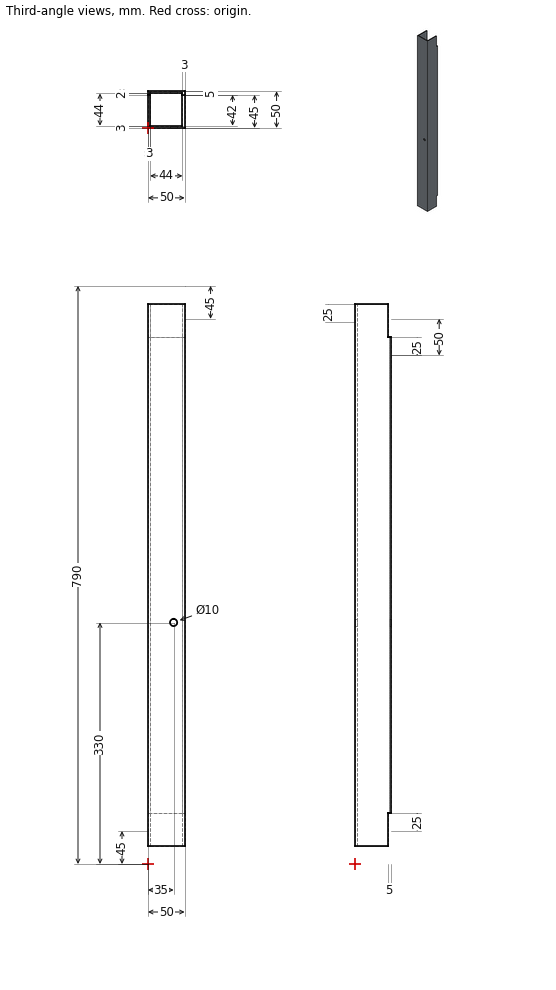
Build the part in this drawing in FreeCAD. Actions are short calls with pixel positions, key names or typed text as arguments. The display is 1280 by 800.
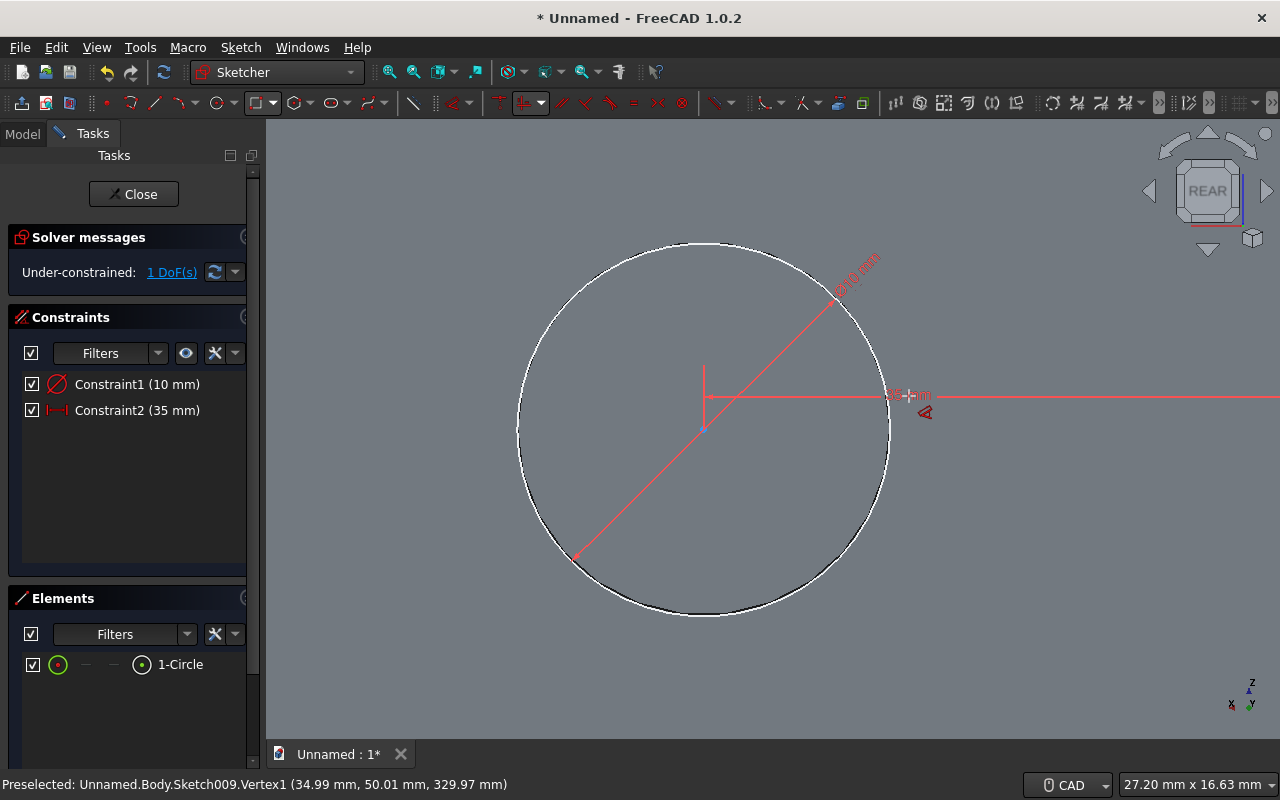
click(704, 430)
click(670, 571)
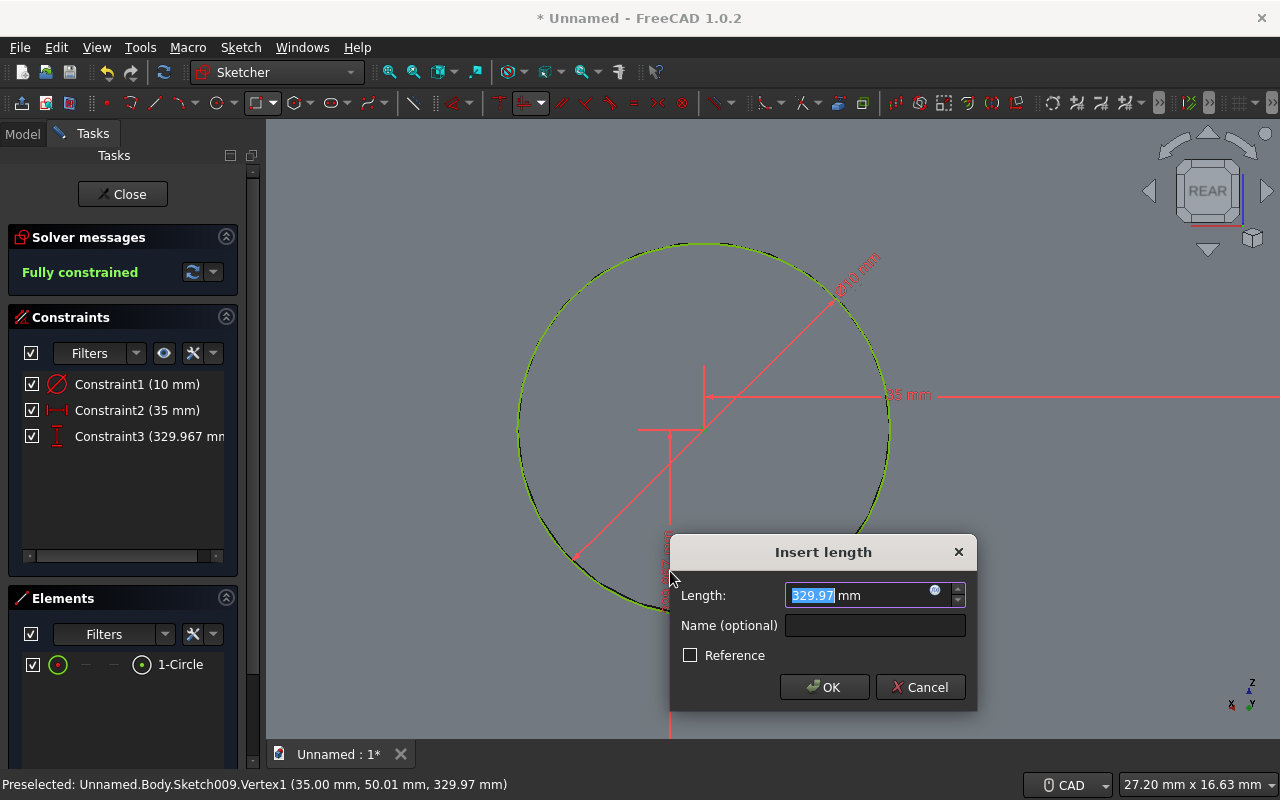
text(330)
key(Return)
key(Escape)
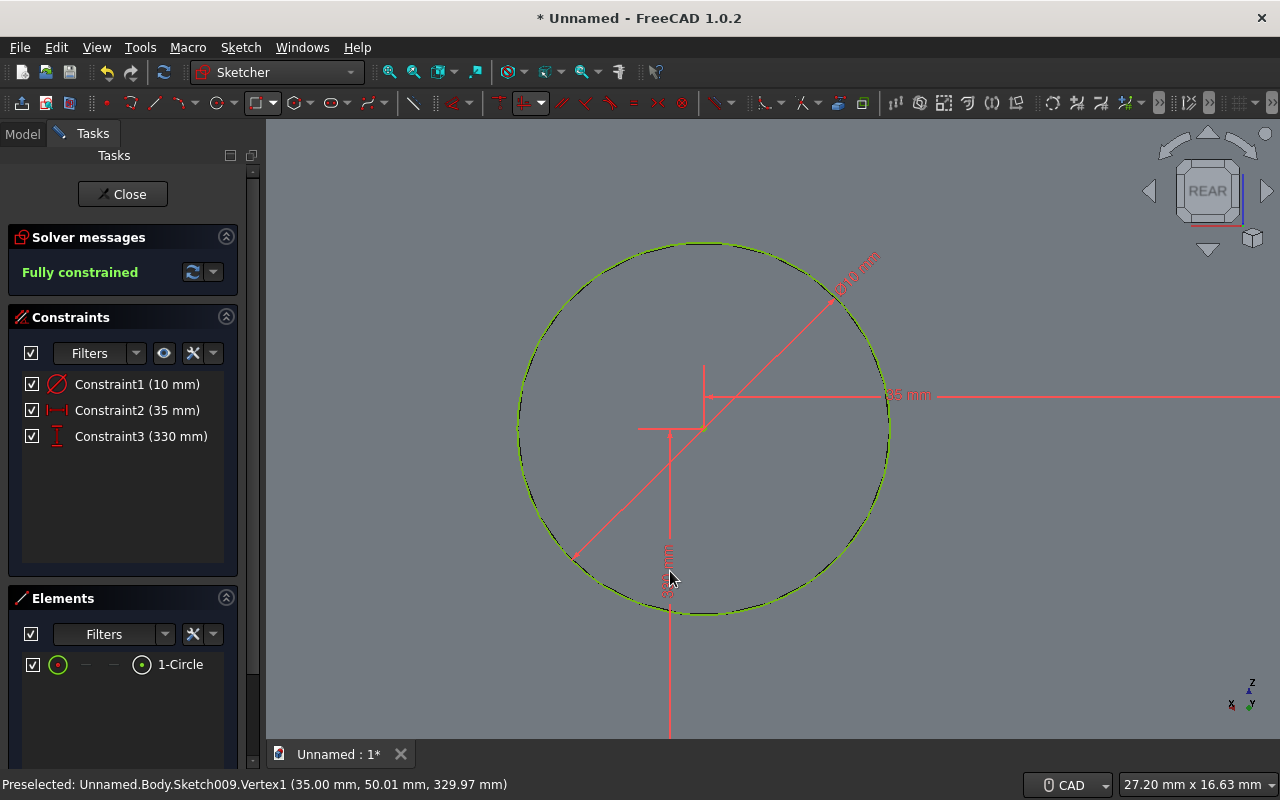
click(123, 194)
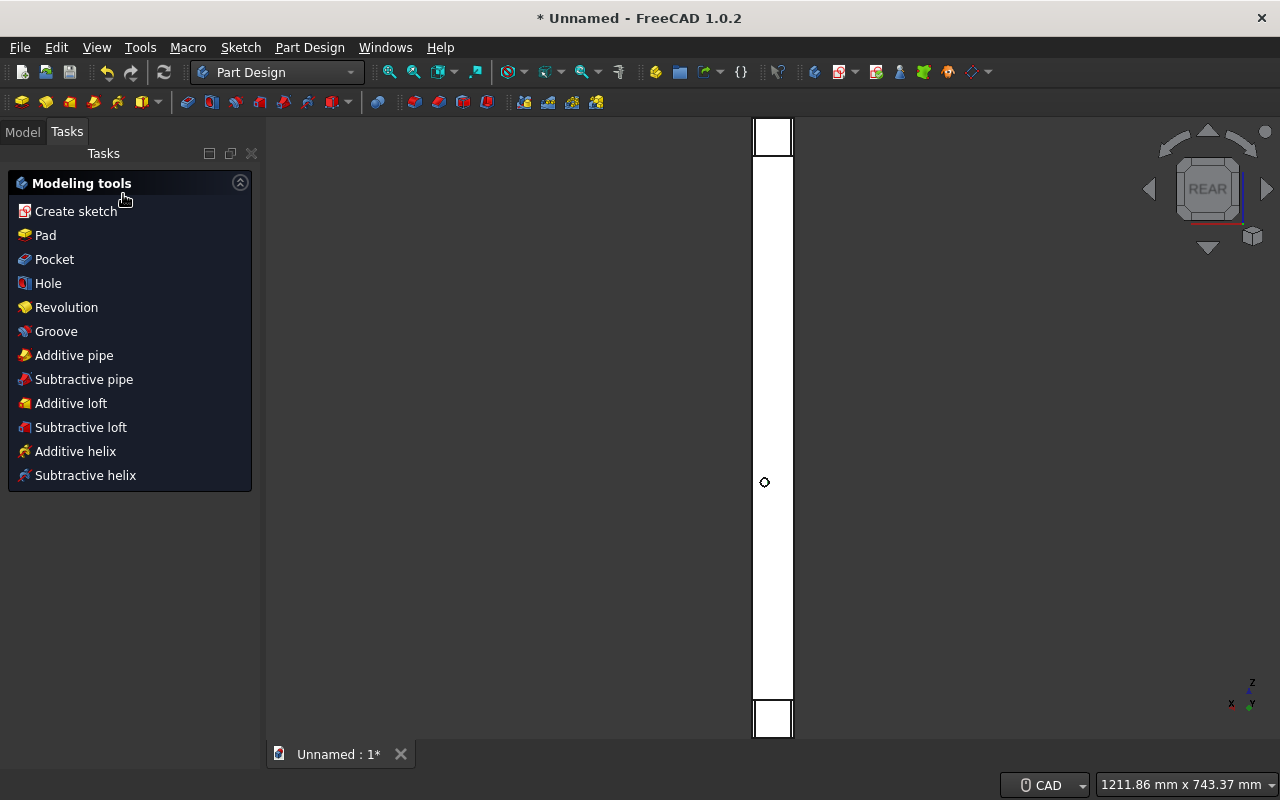
click(188, 102)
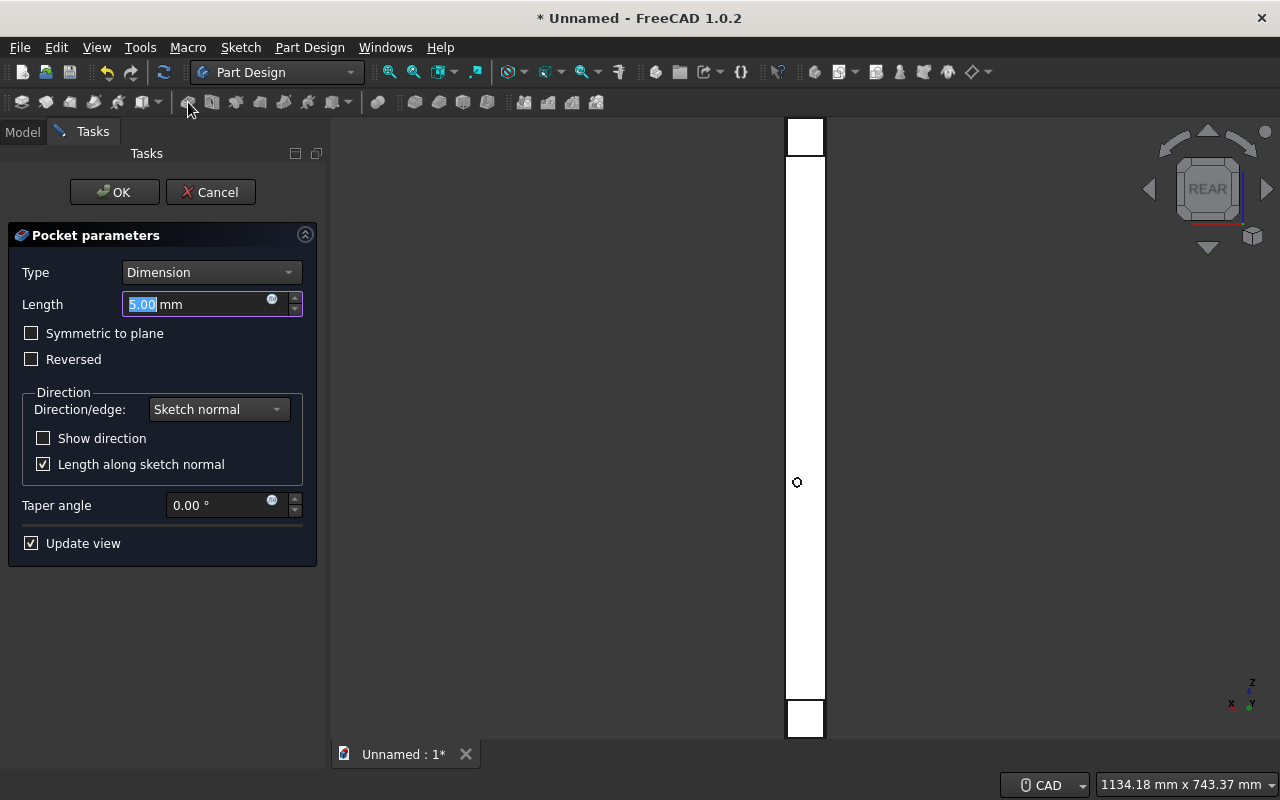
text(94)
key(Tab)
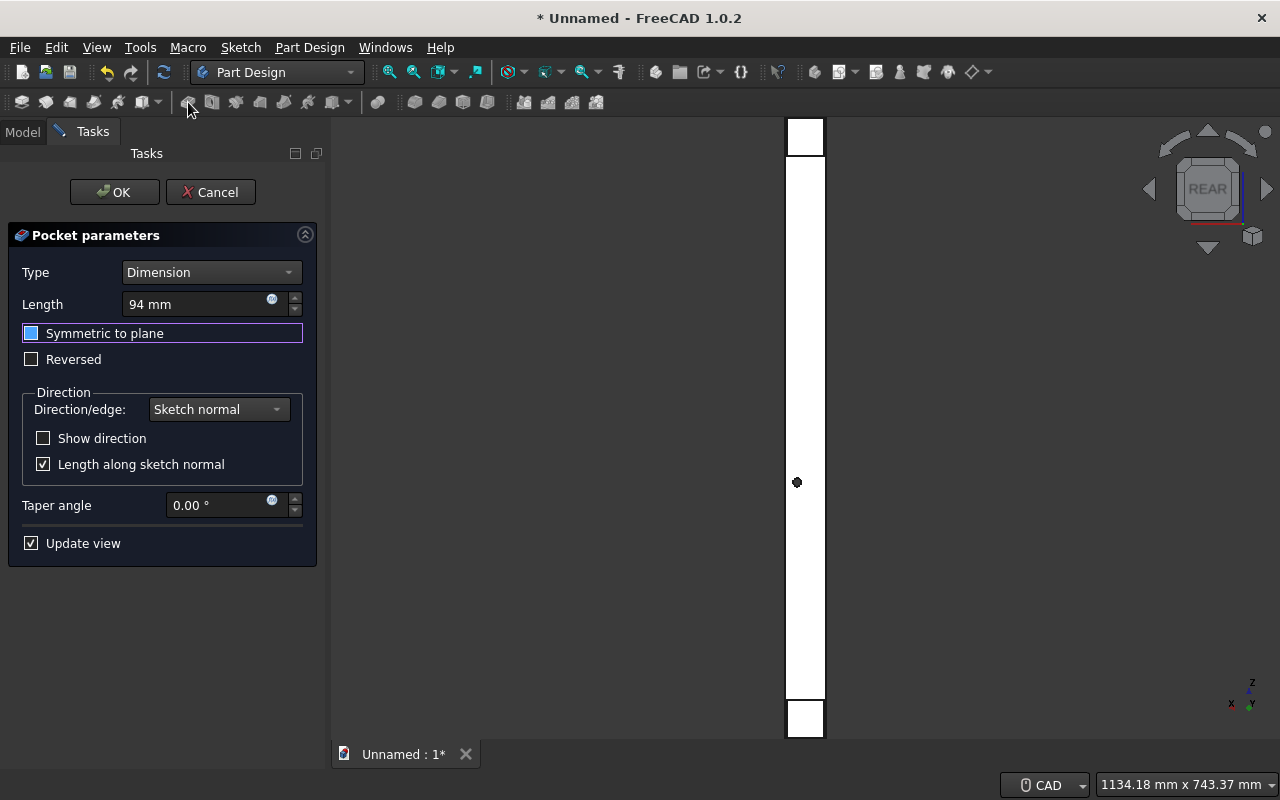
click(115, 192)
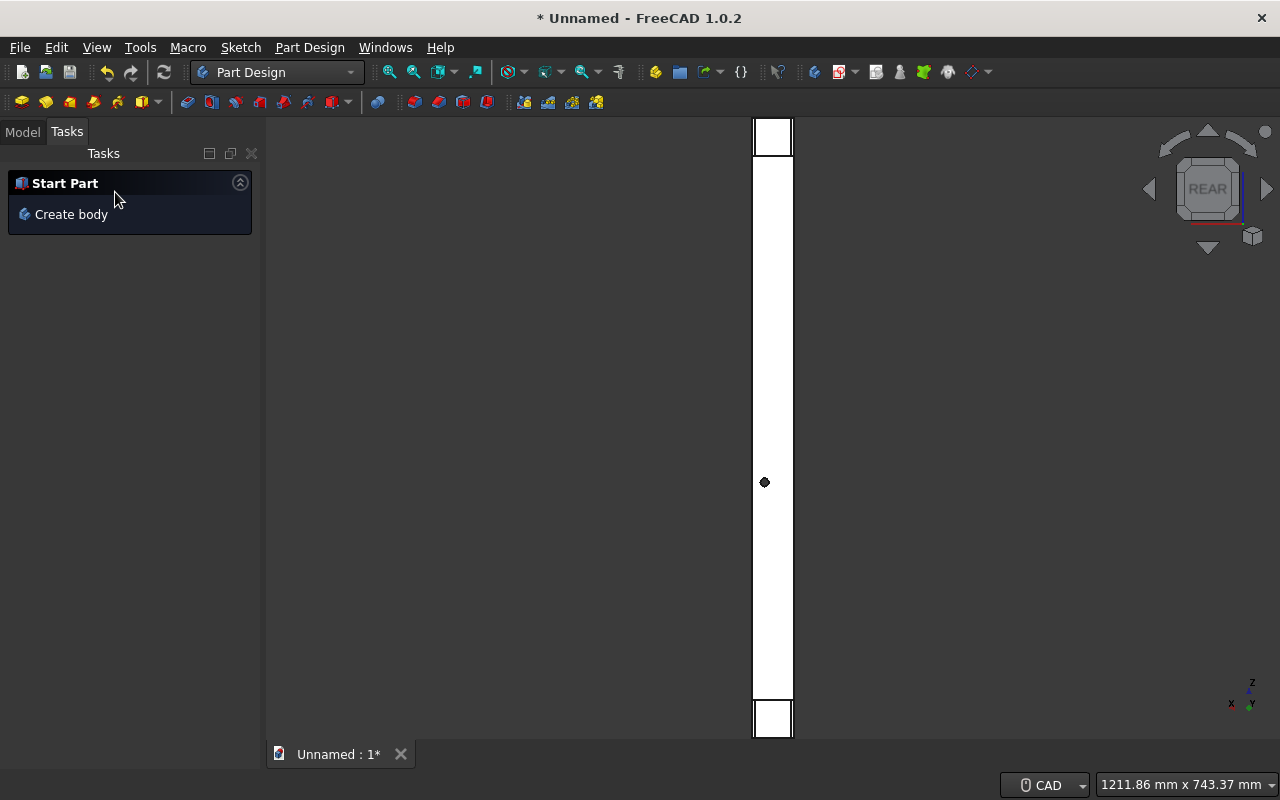
key(0)